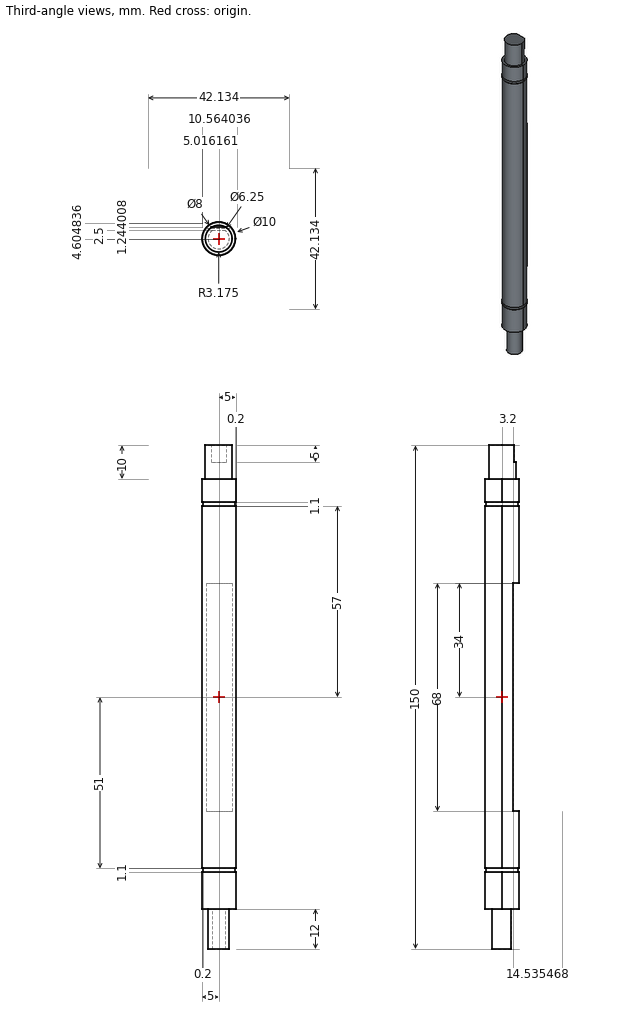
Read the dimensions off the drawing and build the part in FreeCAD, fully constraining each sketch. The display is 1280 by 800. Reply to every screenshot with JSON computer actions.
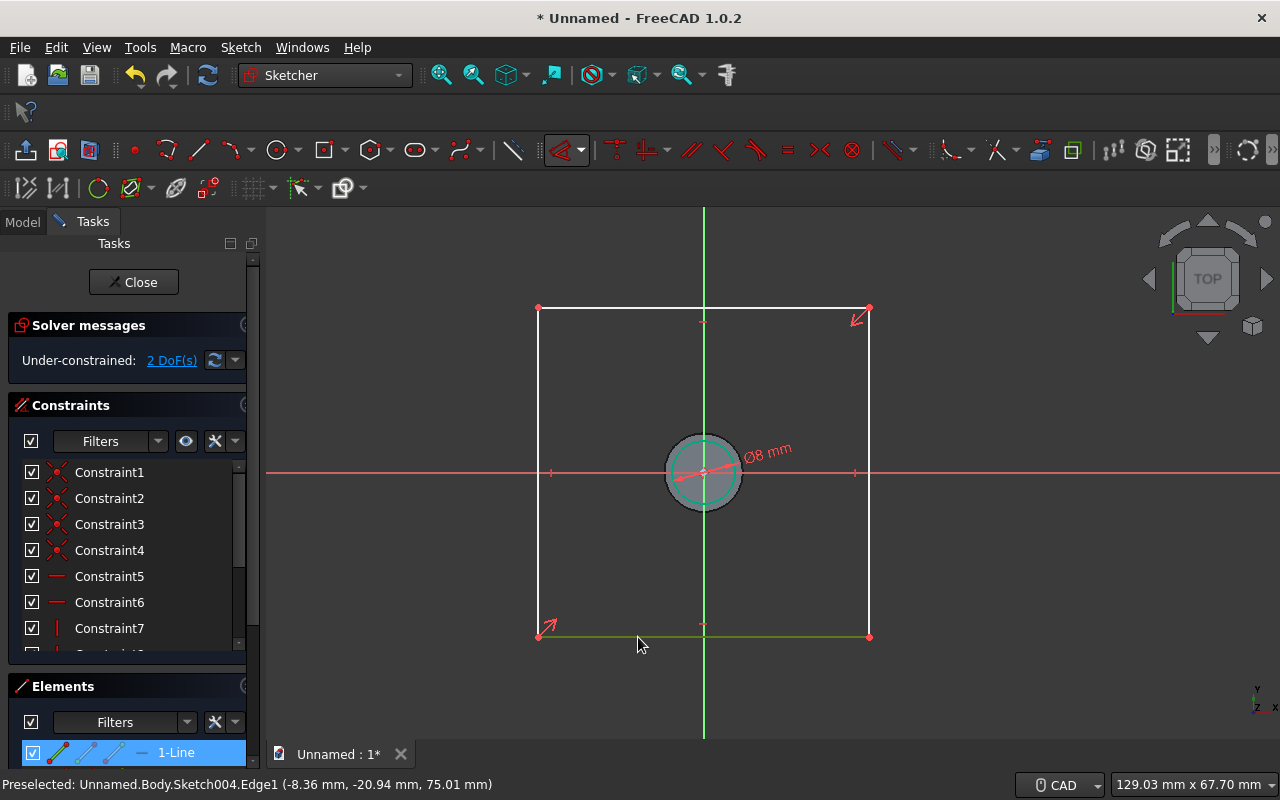
{"action": "key", "text": "l"}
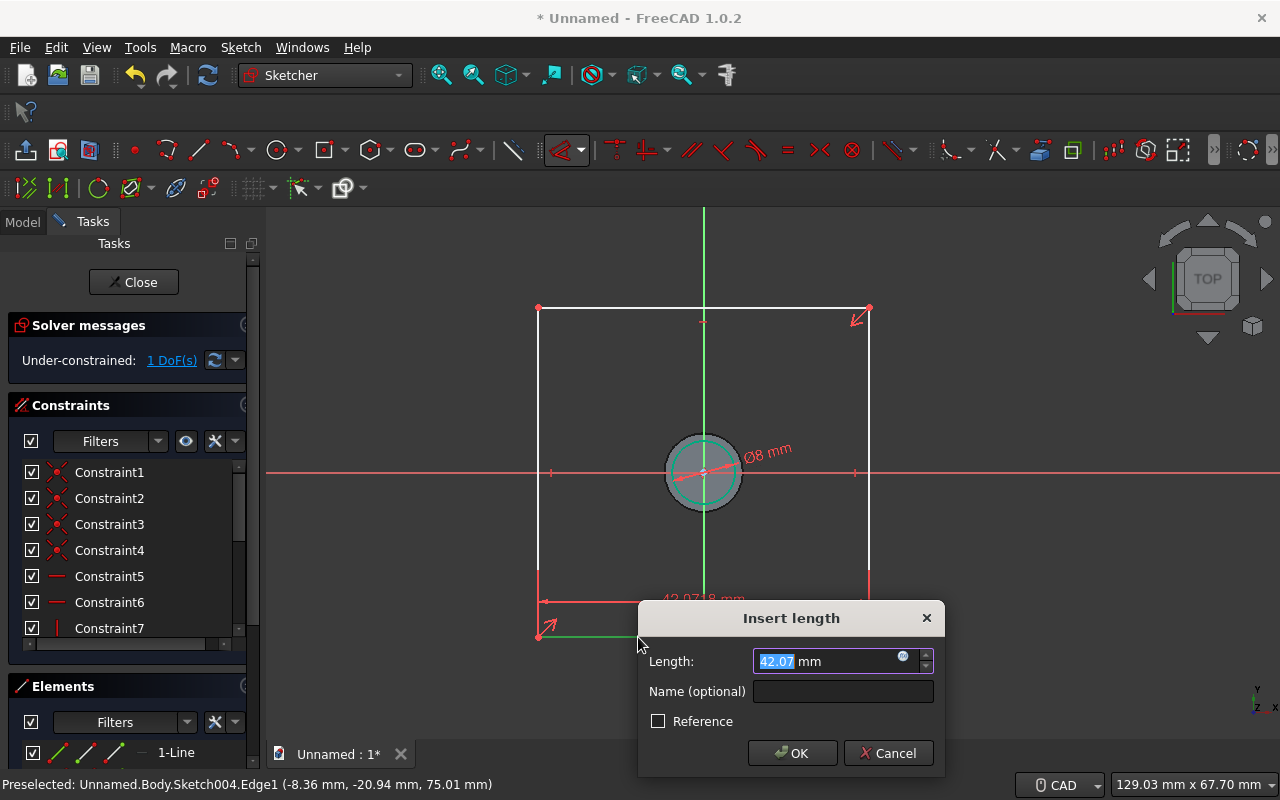
{"action": "type", "text": "42.134"}
{"action": "key", "text": "Return"}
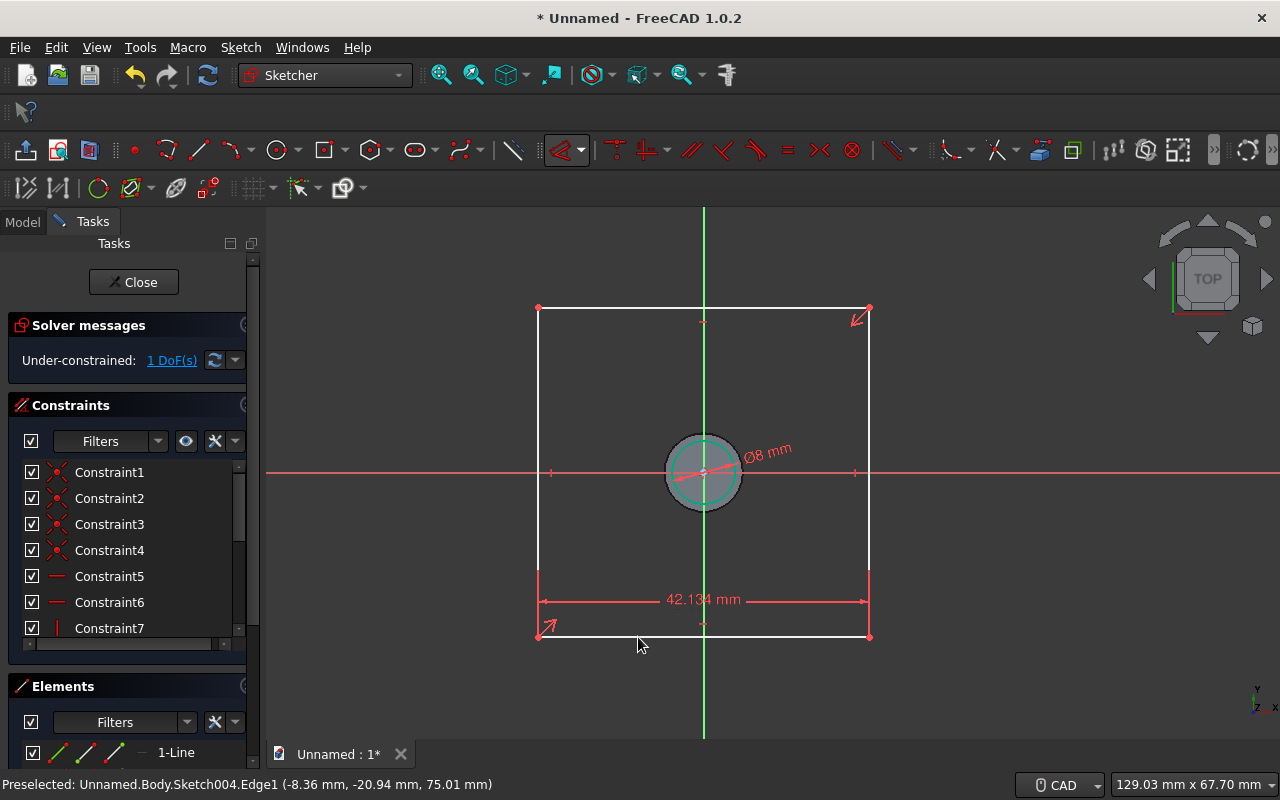
{"action": "left_click", "coordinate": [869, 538]}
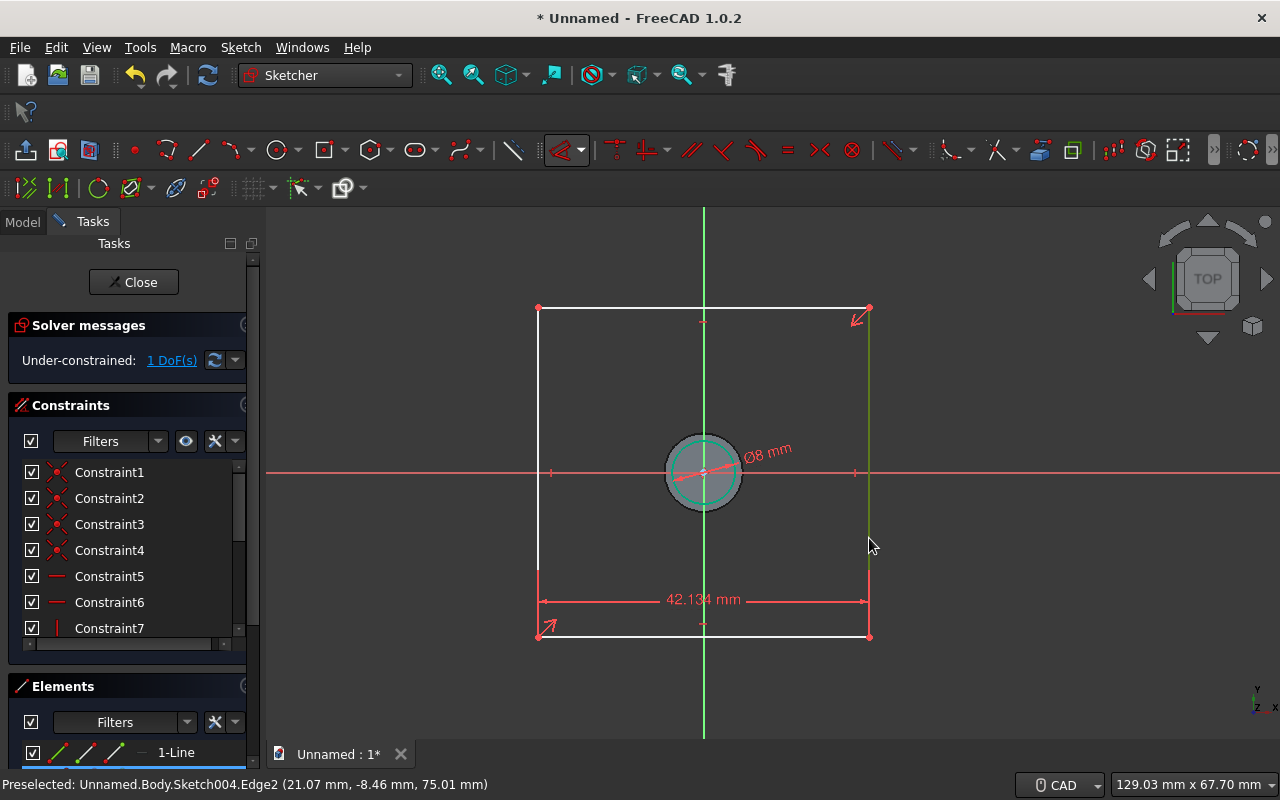
{"action": "left_click", "coordinate": [584, 150]}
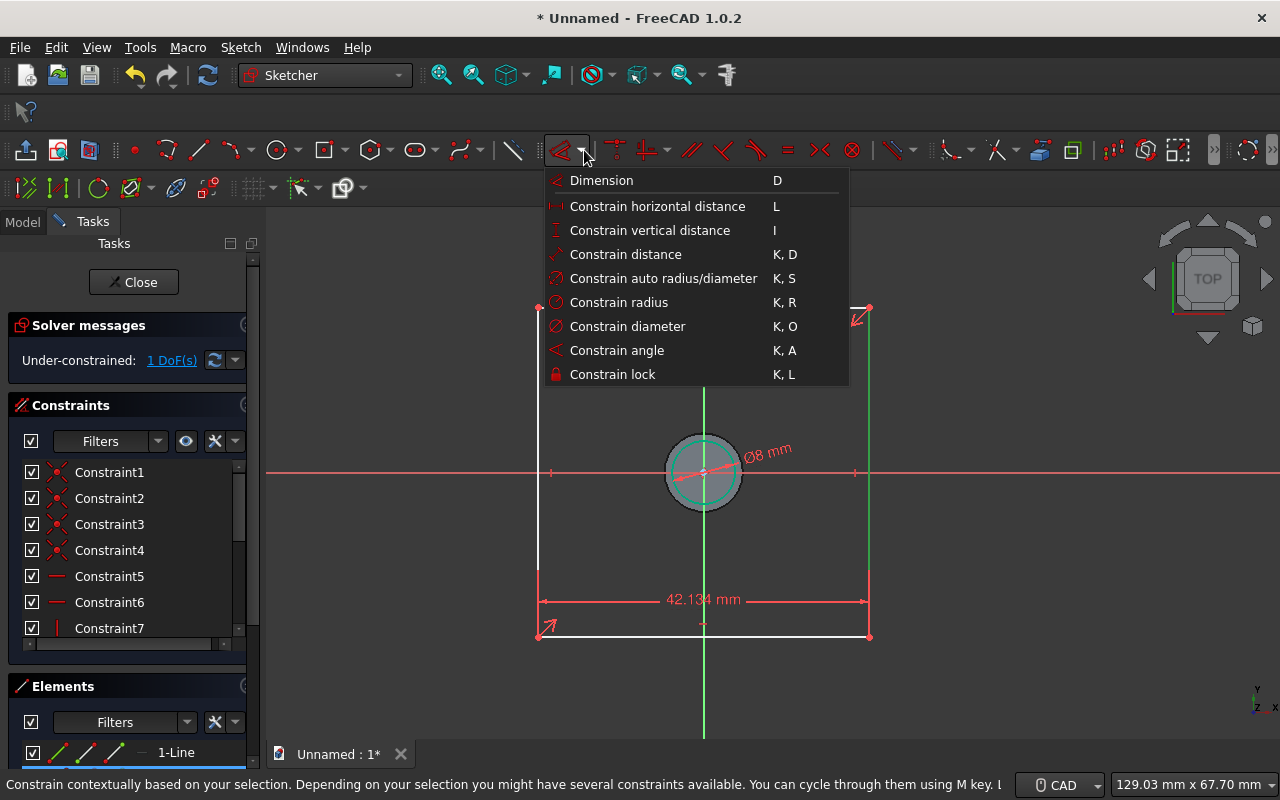
{"action": "left_click", "coordinate": [697, 230]}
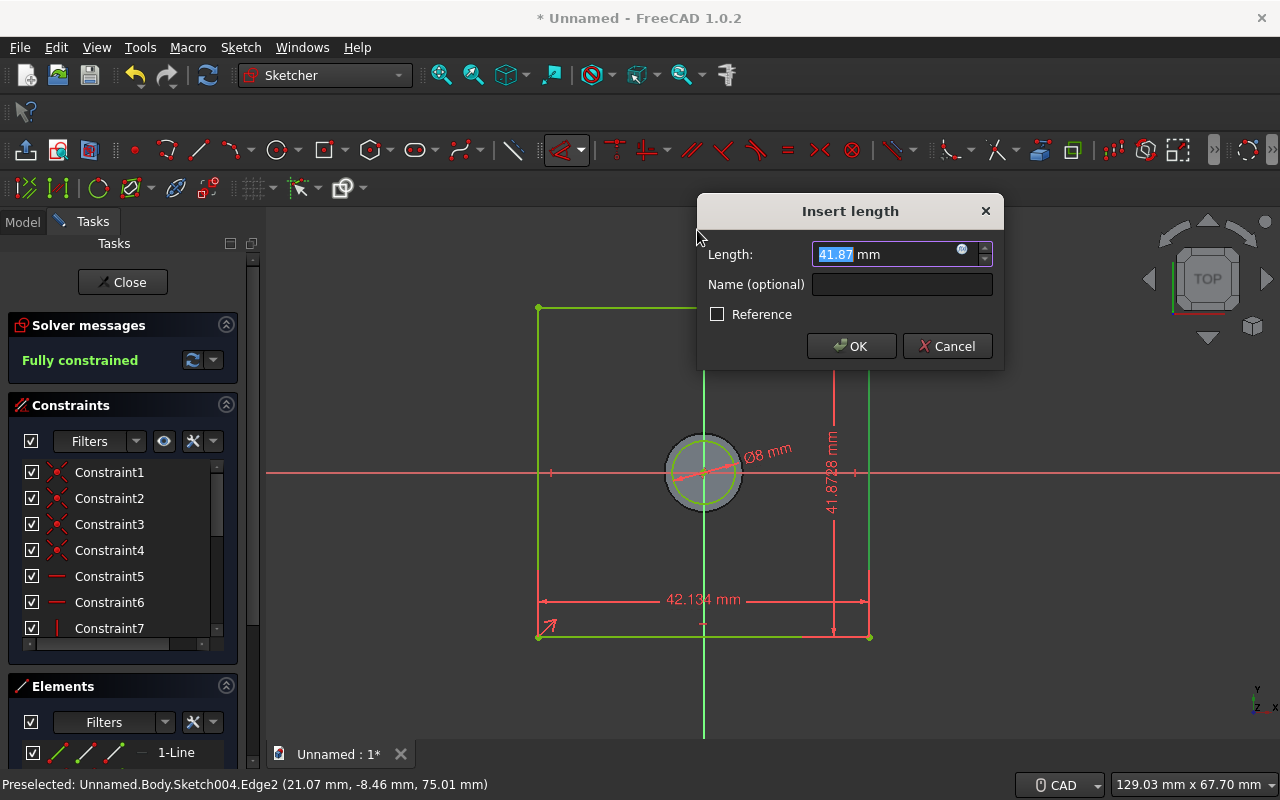
{"action": "type", "text": "42.134"}
{"action": "key", "text": "Return"}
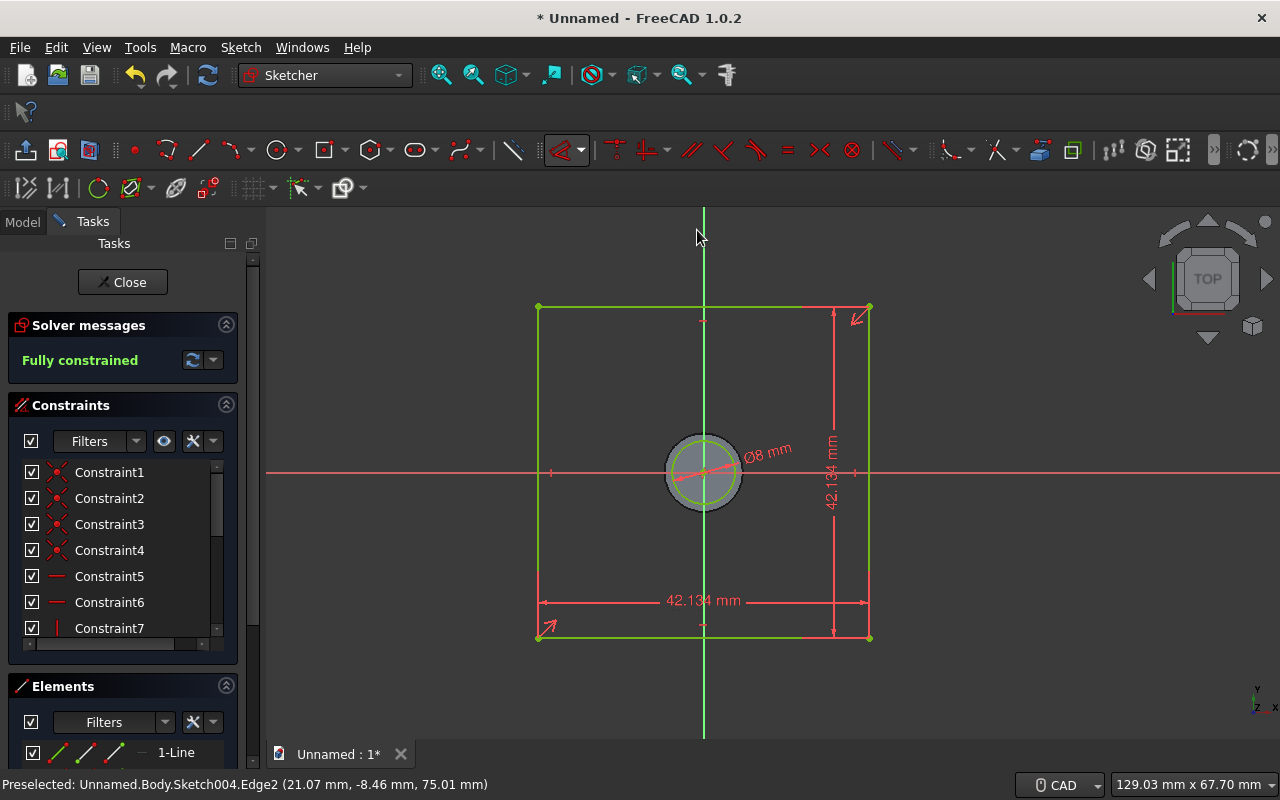
{"action": "left_click", "coordinate": [123, 282]}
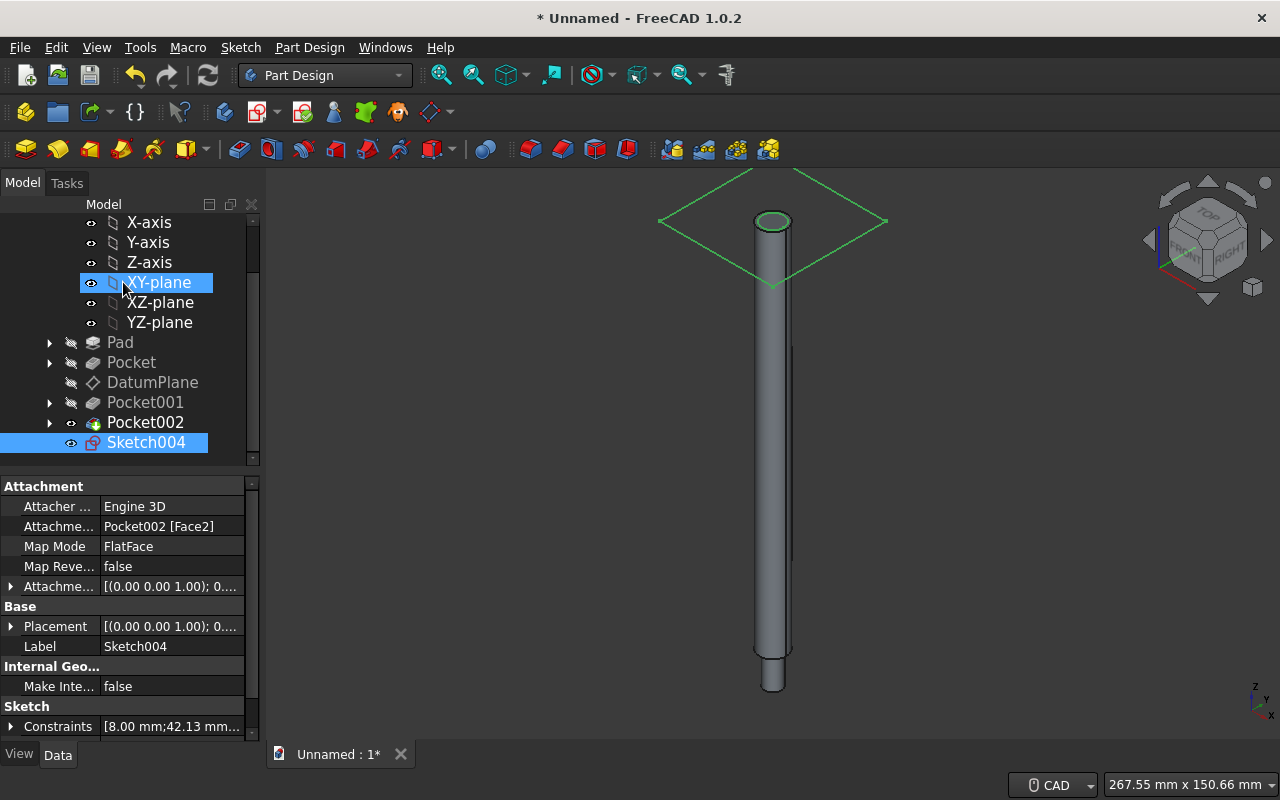
{"action": "left_click", "coordinate": [240, 150]}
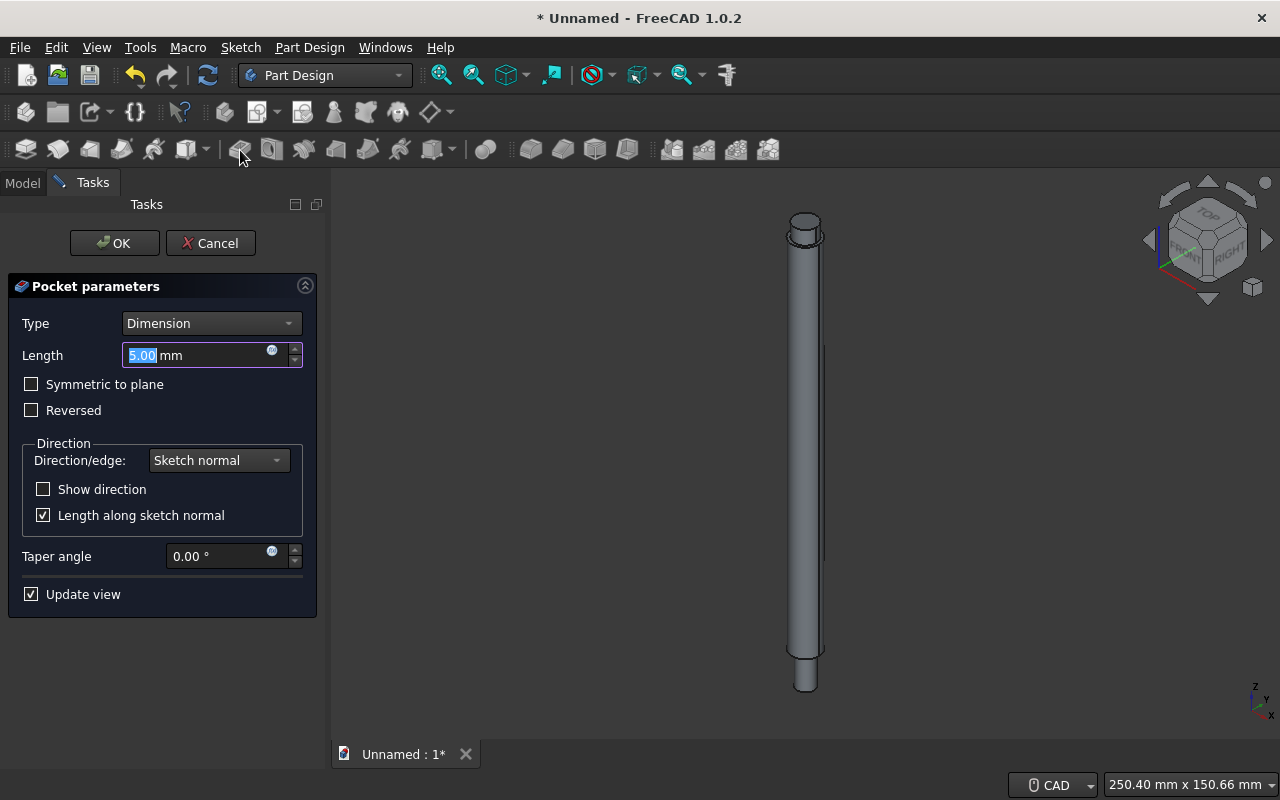
{"action": "type", "text": "10"}
{"action": "key", "text": "Tab"}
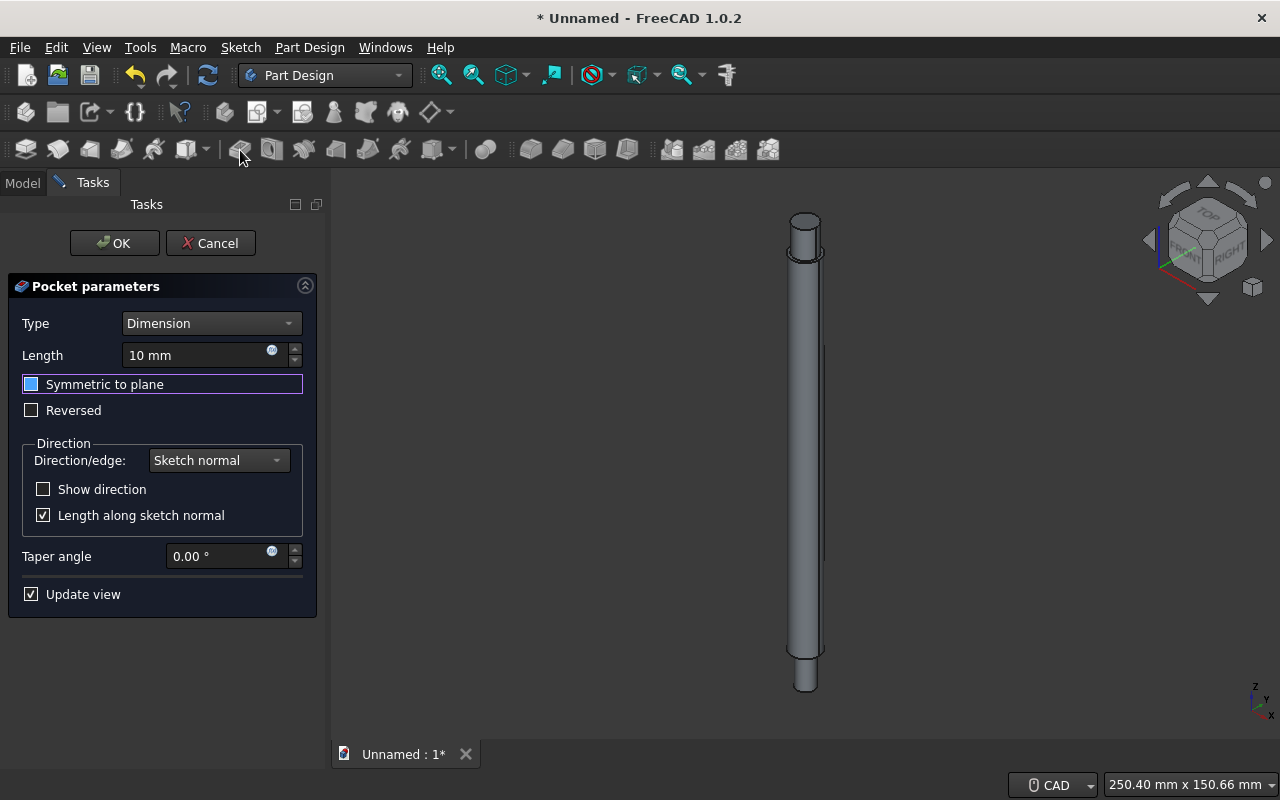
{"action": "left_click", "coordinate": [115, 243]}